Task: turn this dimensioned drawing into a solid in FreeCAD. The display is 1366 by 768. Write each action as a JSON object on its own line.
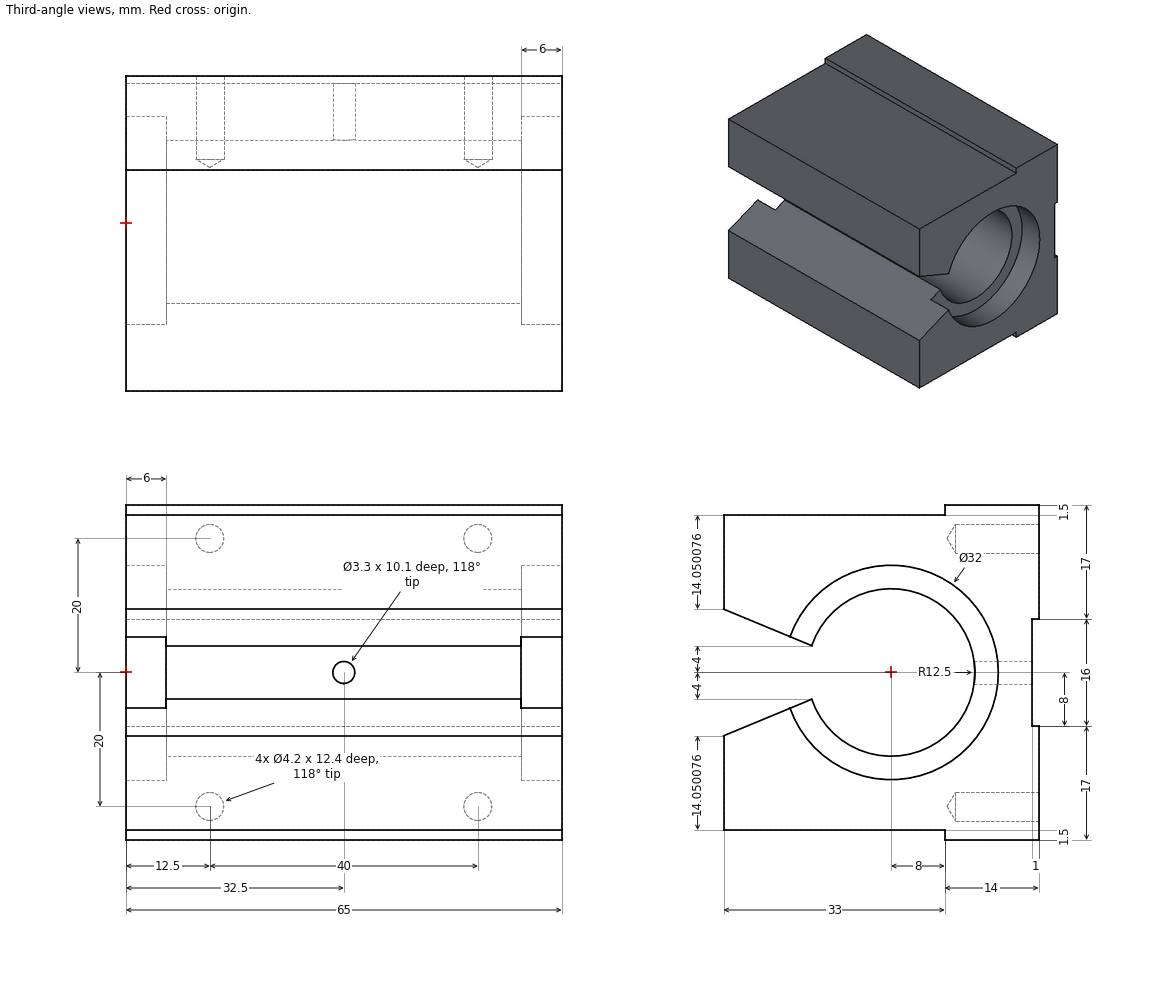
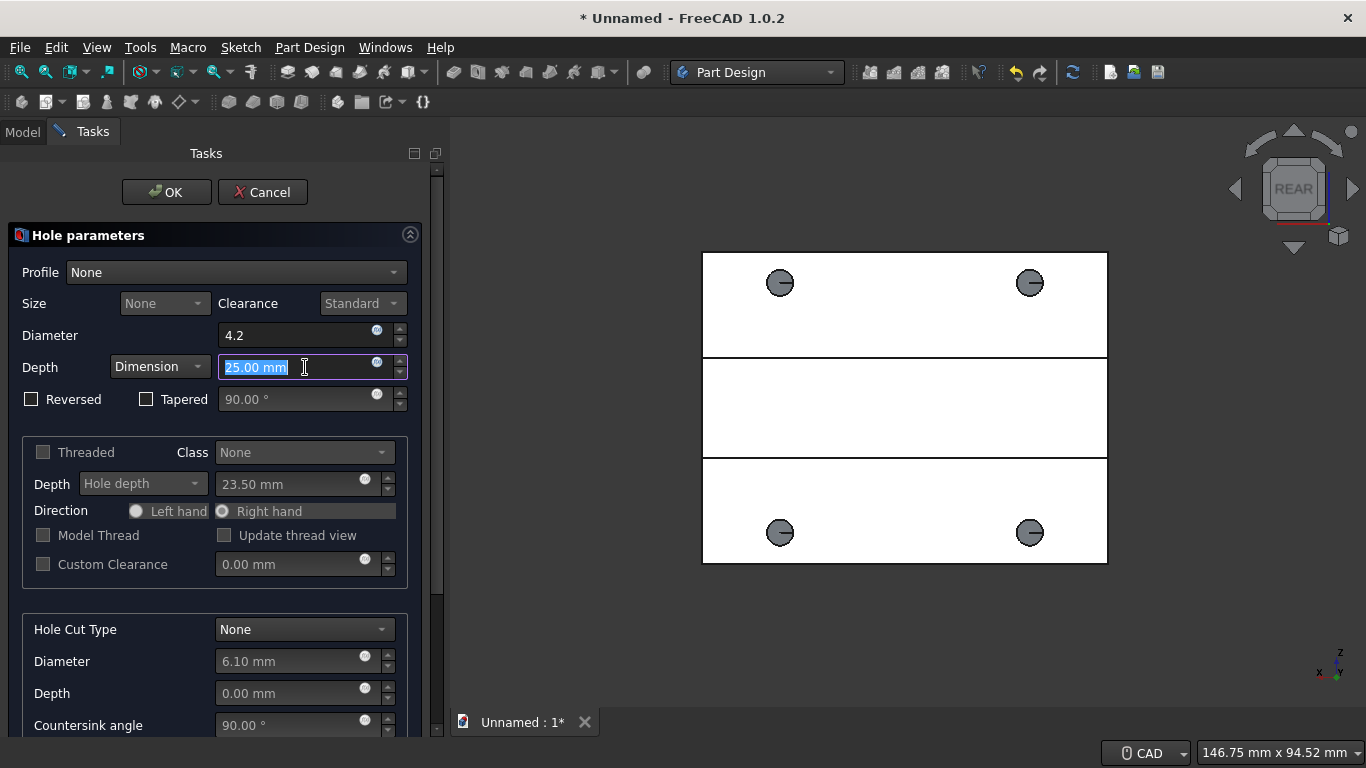
{"action": "type", "text": "12.4"}
{"action": "key", "text": "Tab"}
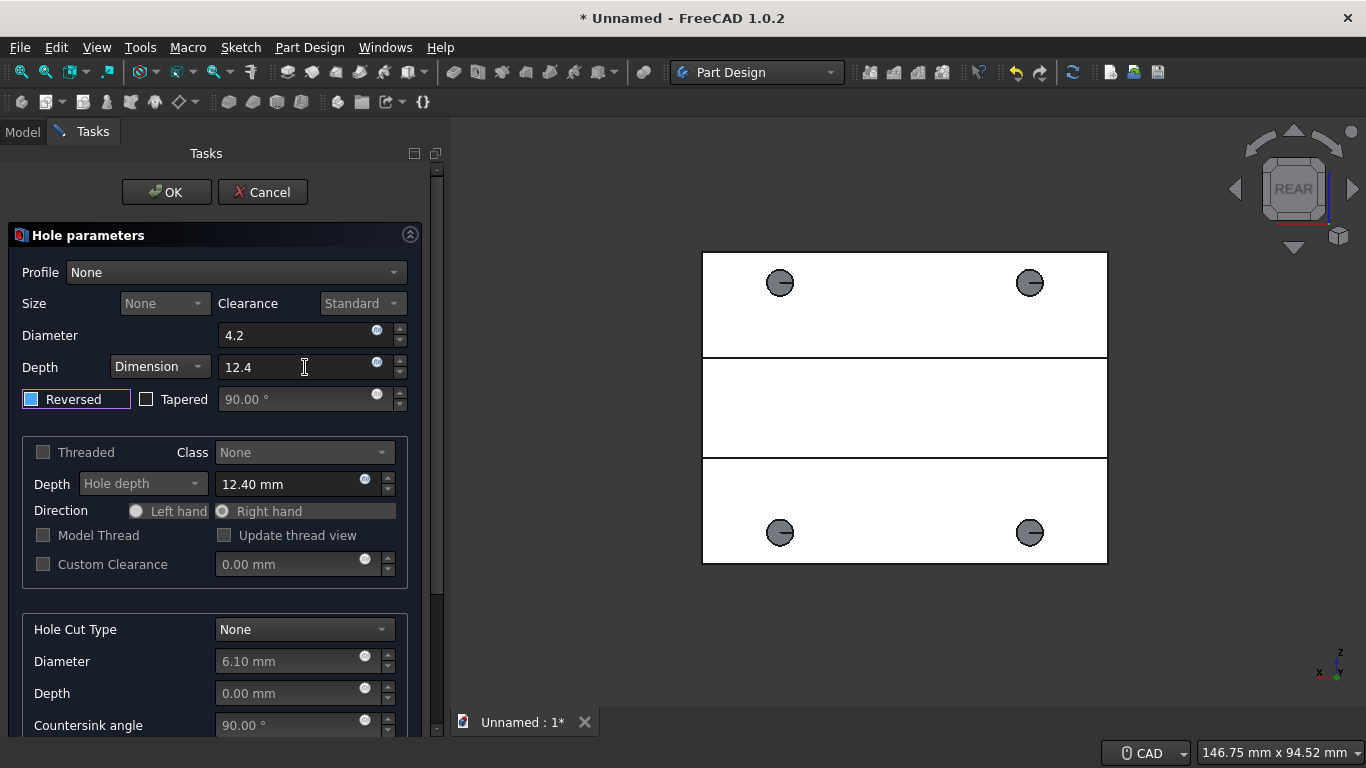
{"action": "left_click", "coordinate": [167, 192]}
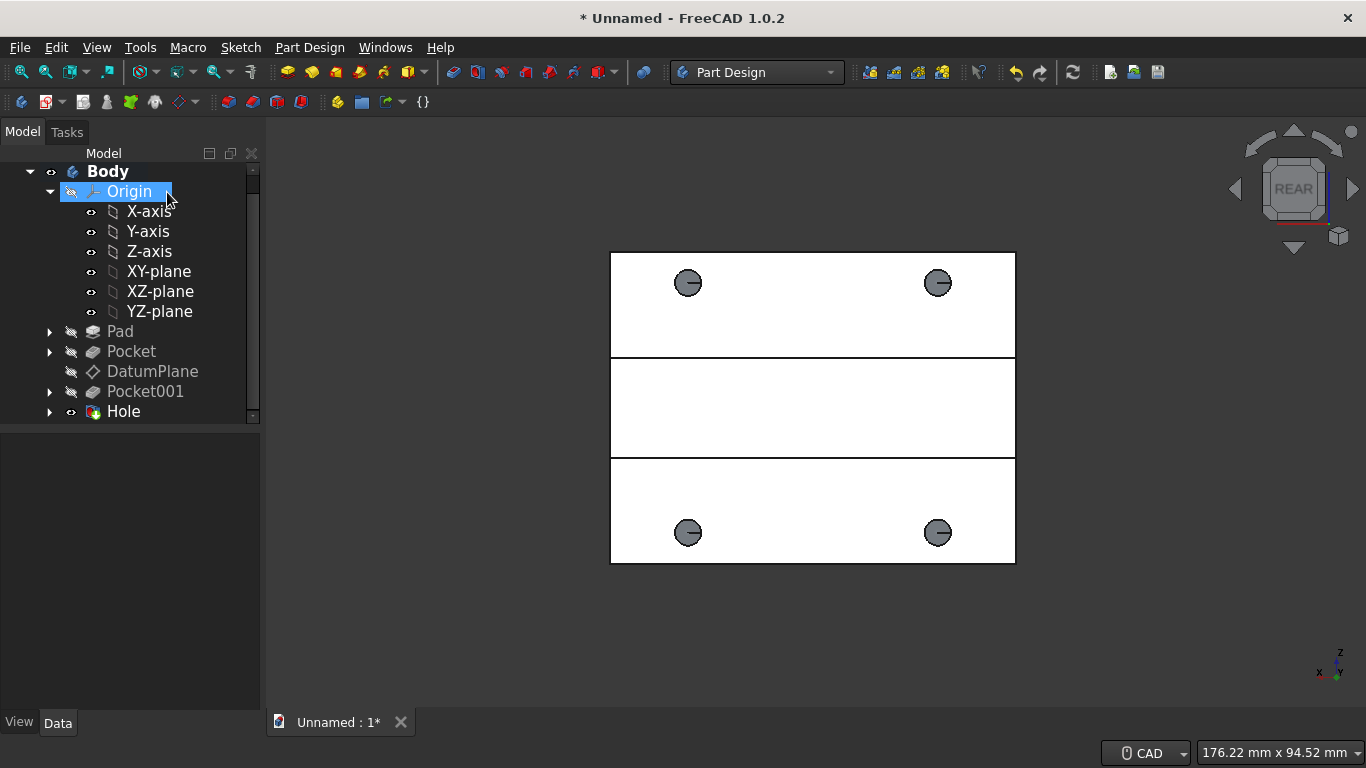
{"action": "left_click", "coordinate": [813, 304]}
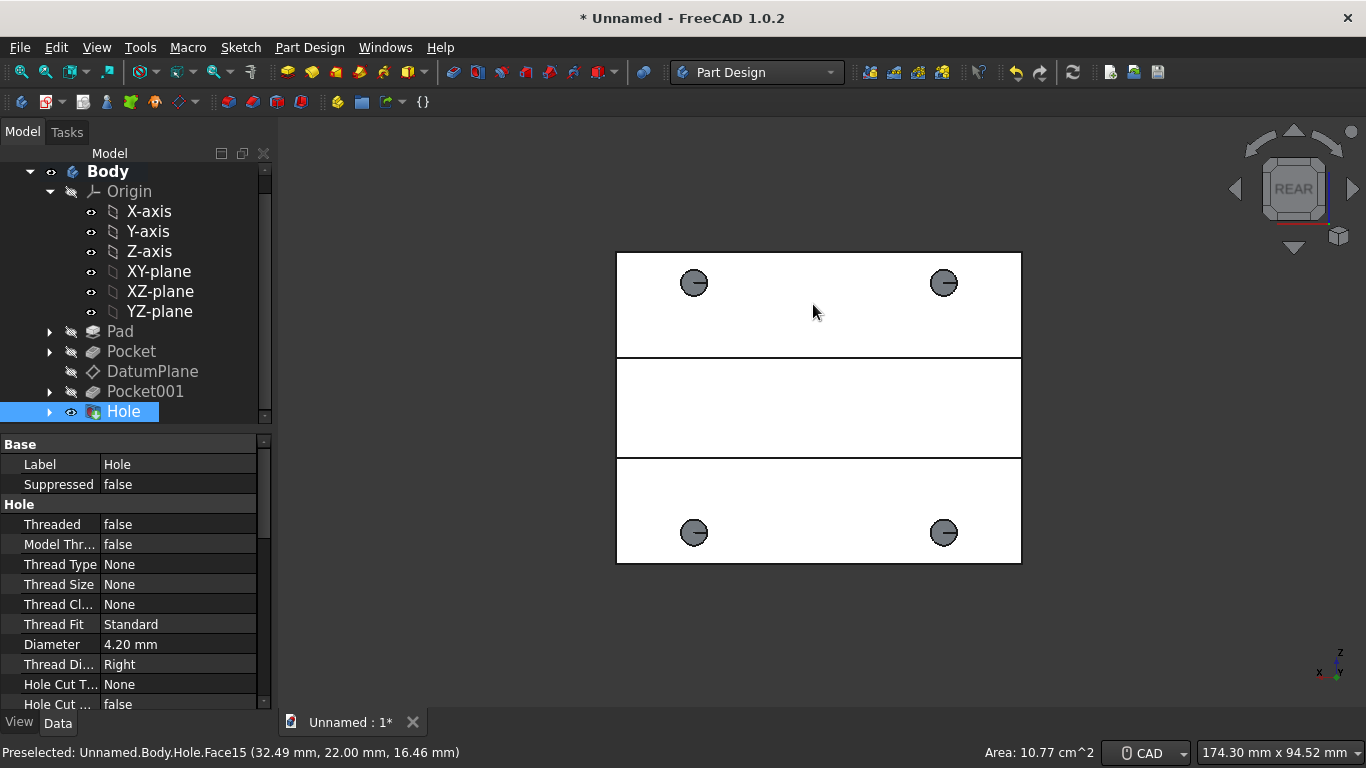
{"action": "left_click", "coordinate": [46, 102]}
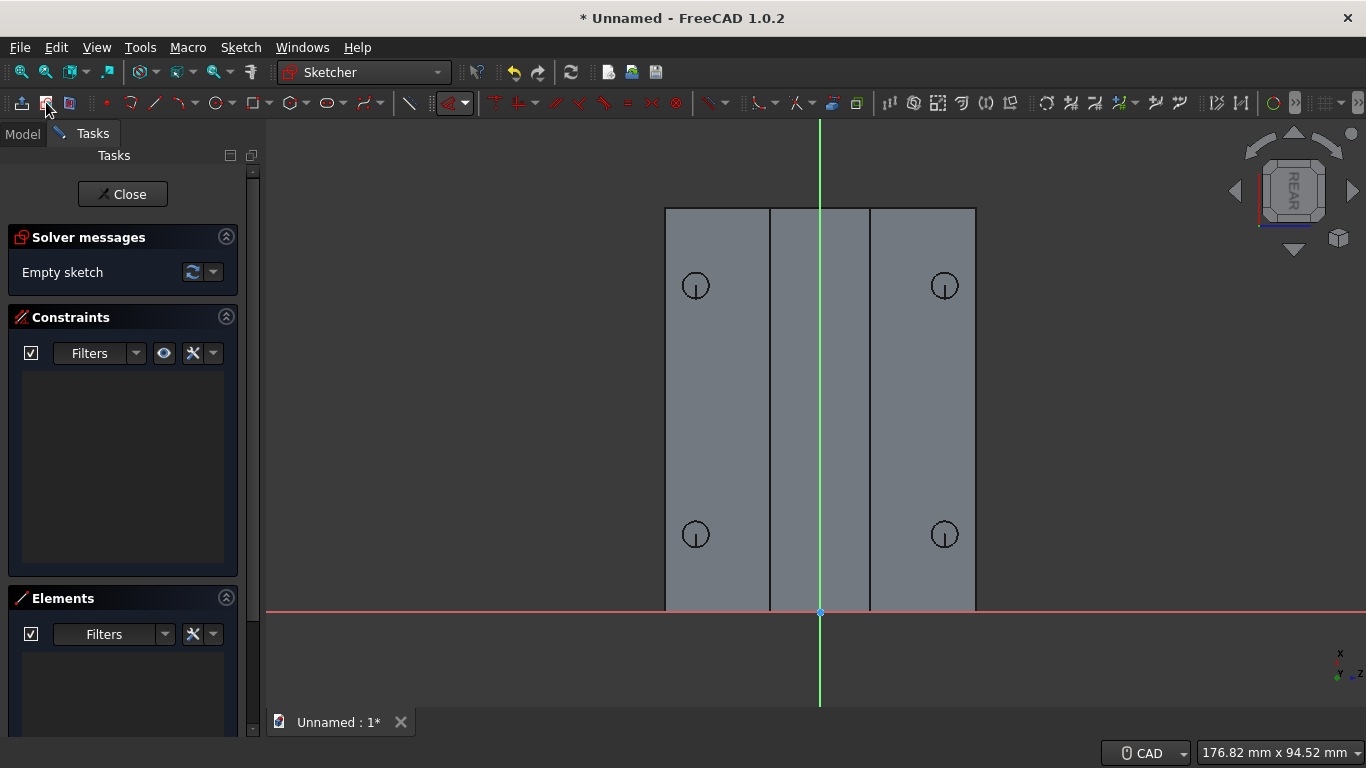
{"action": "scroll", "coordinate": [824, 410], "scroll_direction": "up", "scroll_amount": 15}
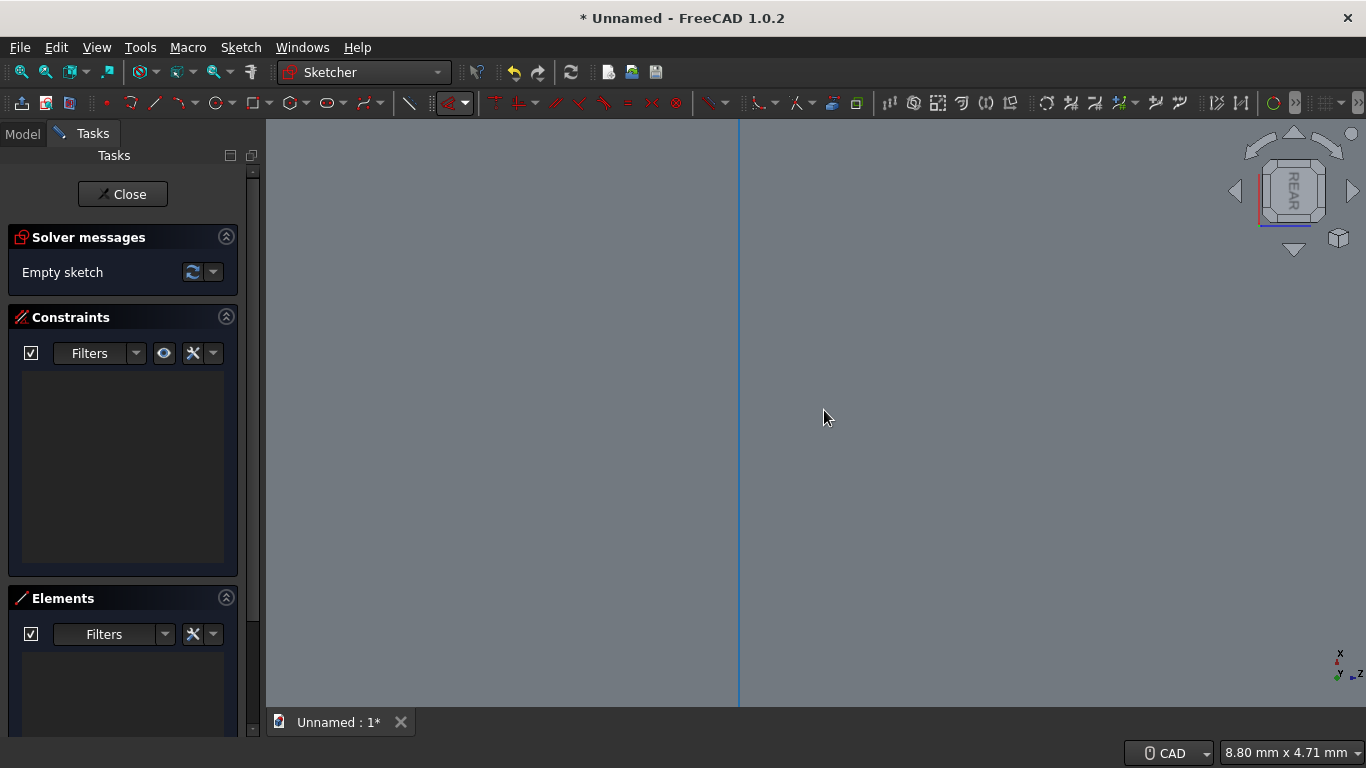
{"action": "left_click", "coordinate": [216, 104]}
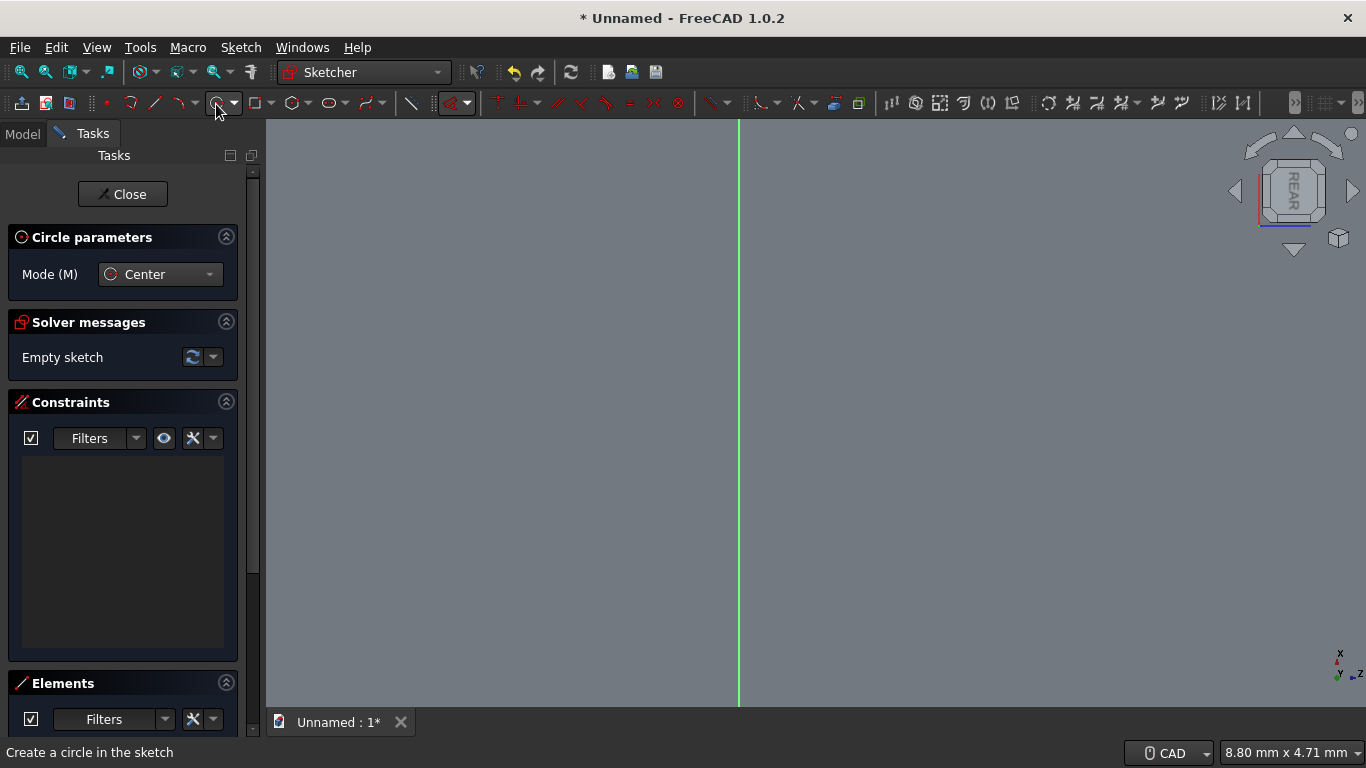
{"action": "left_click", "coordinate": [739, 400]}
{"action": "left_click", "coordinate": [885, 254]}
{"action": "key", "text": "Escape"}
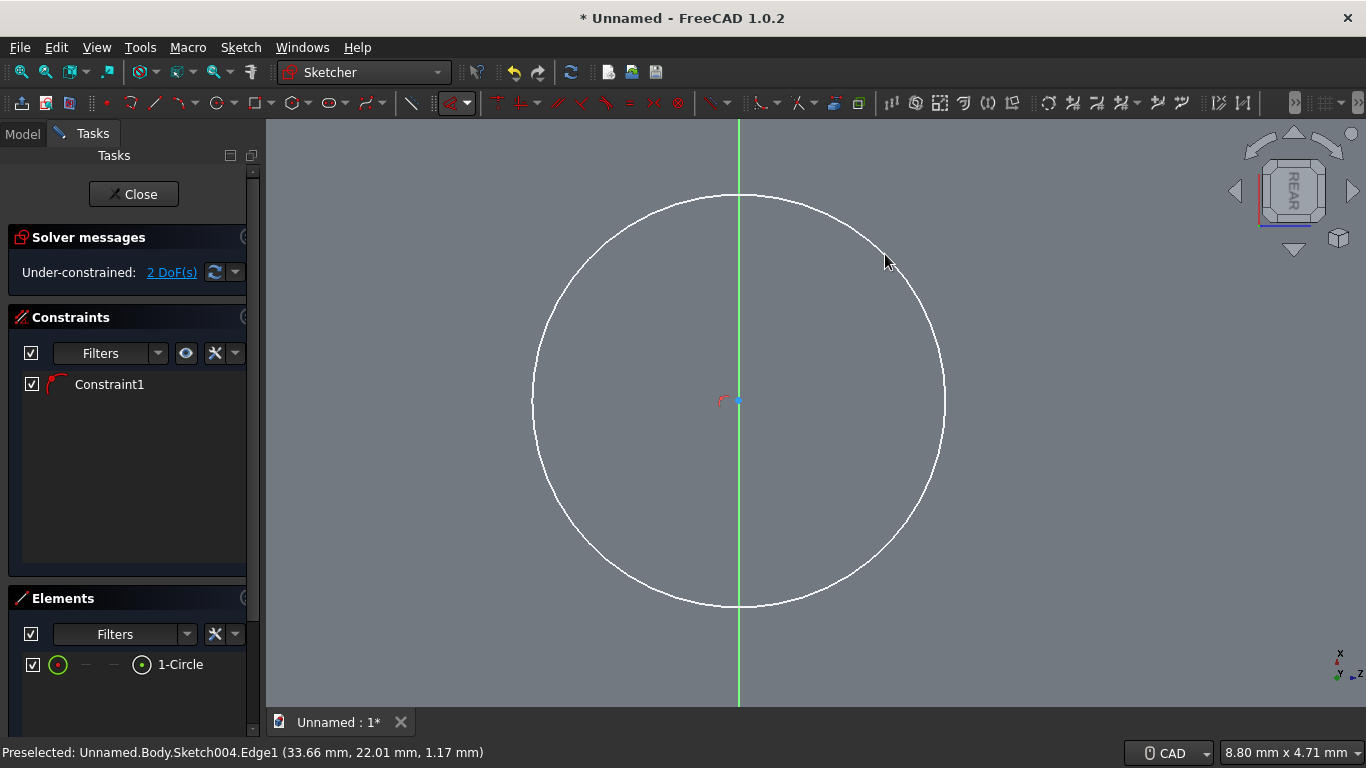
{"action": "left_click", "coordinate": [884, 254]}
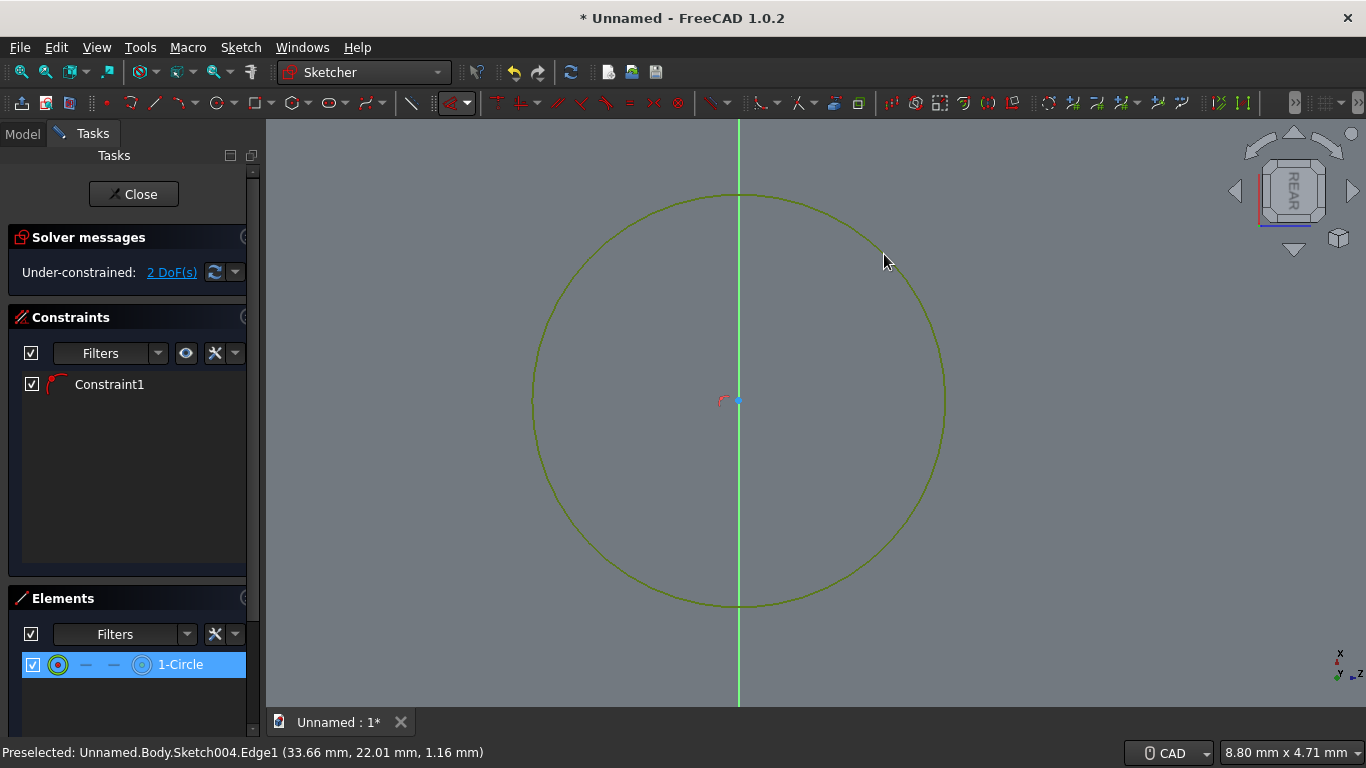
{"action": "key", "text": "k o"}